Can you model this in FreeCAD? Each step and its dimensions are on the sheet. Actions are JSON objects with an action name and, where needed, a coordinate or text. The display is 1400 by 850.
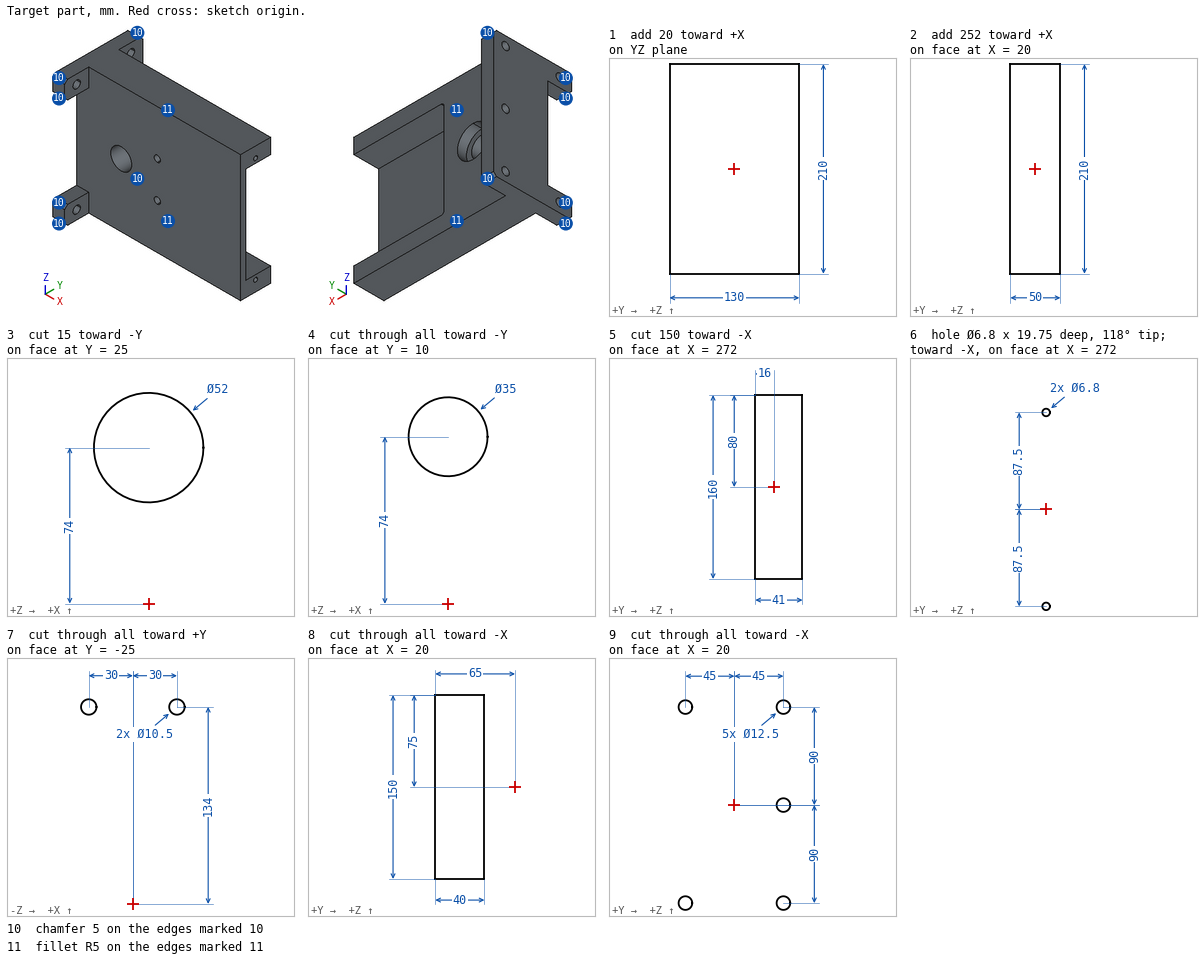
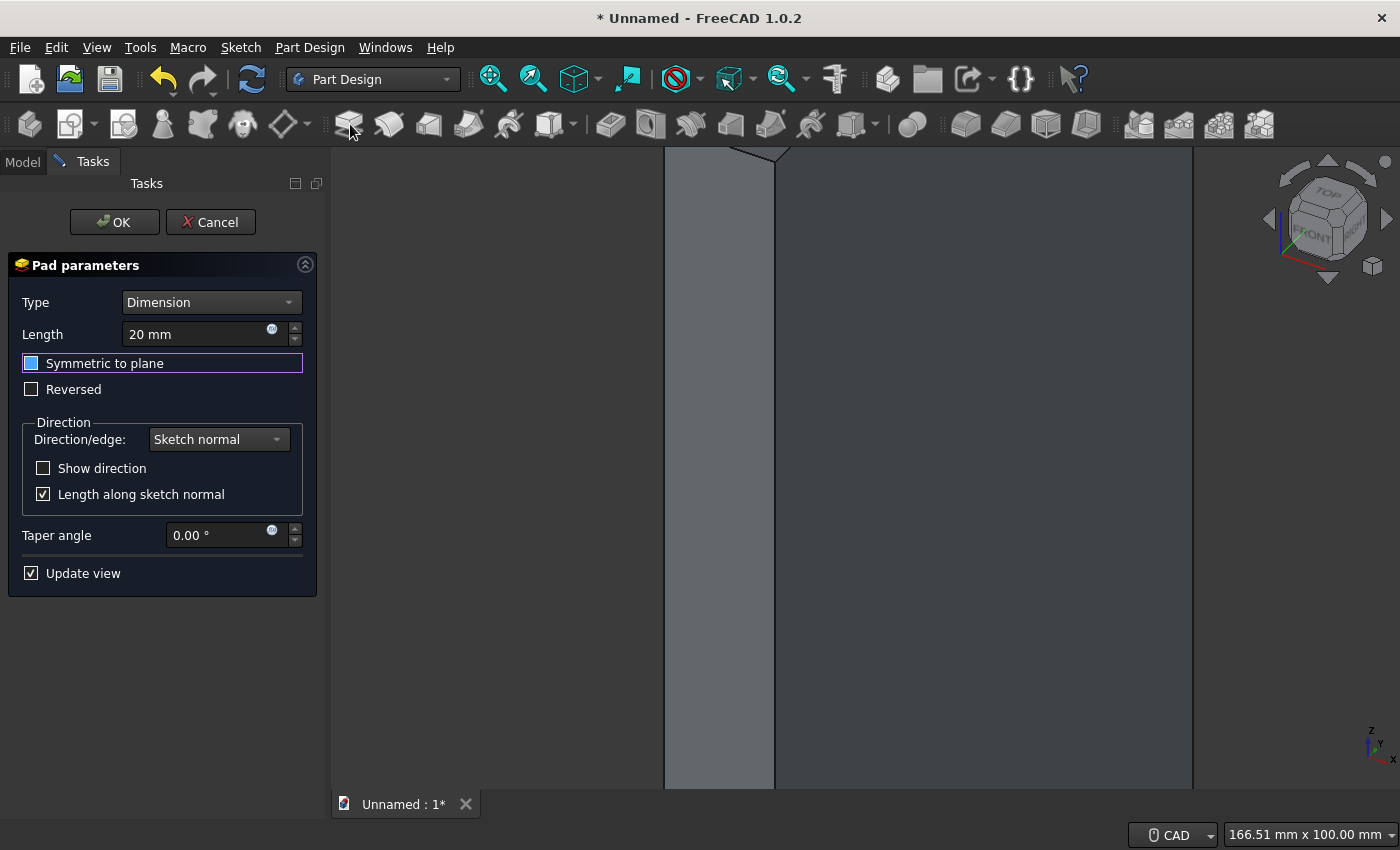
{"action": "left_click", "coordinate": [115, 222]}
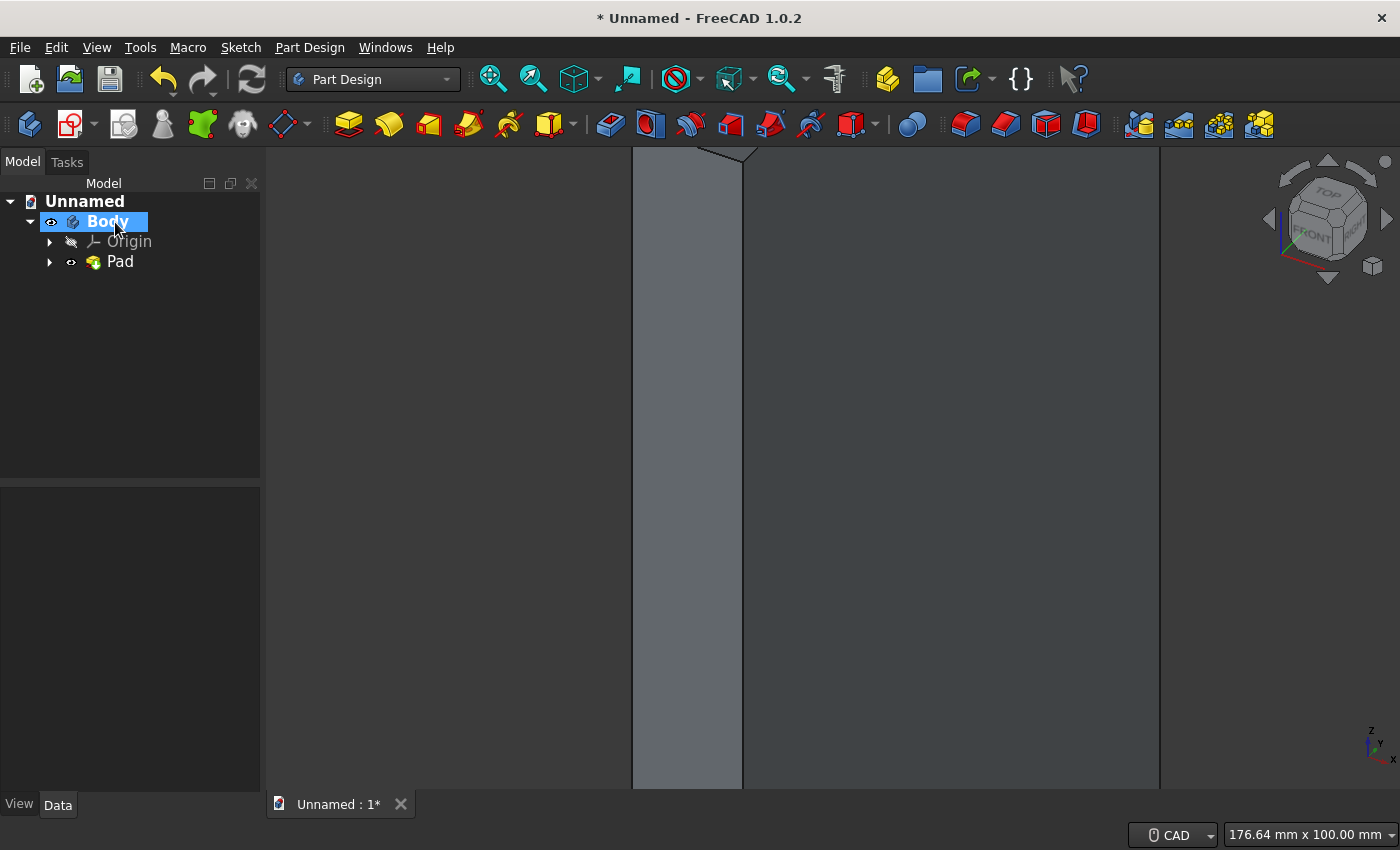
{"action": "left_click", "coordinate": [494, 80]}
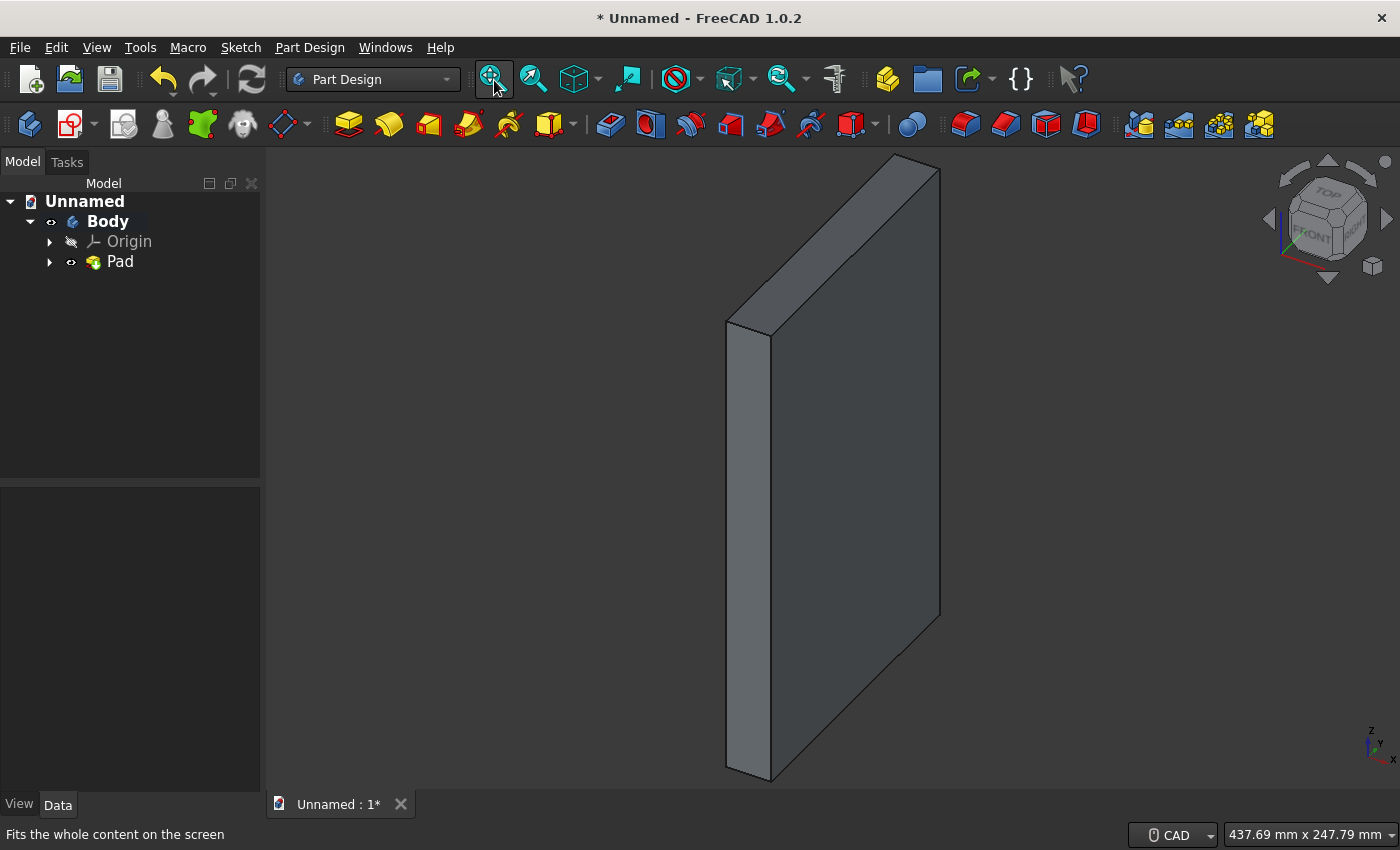
{"action": "left_click", "coordinate": [855, 474]}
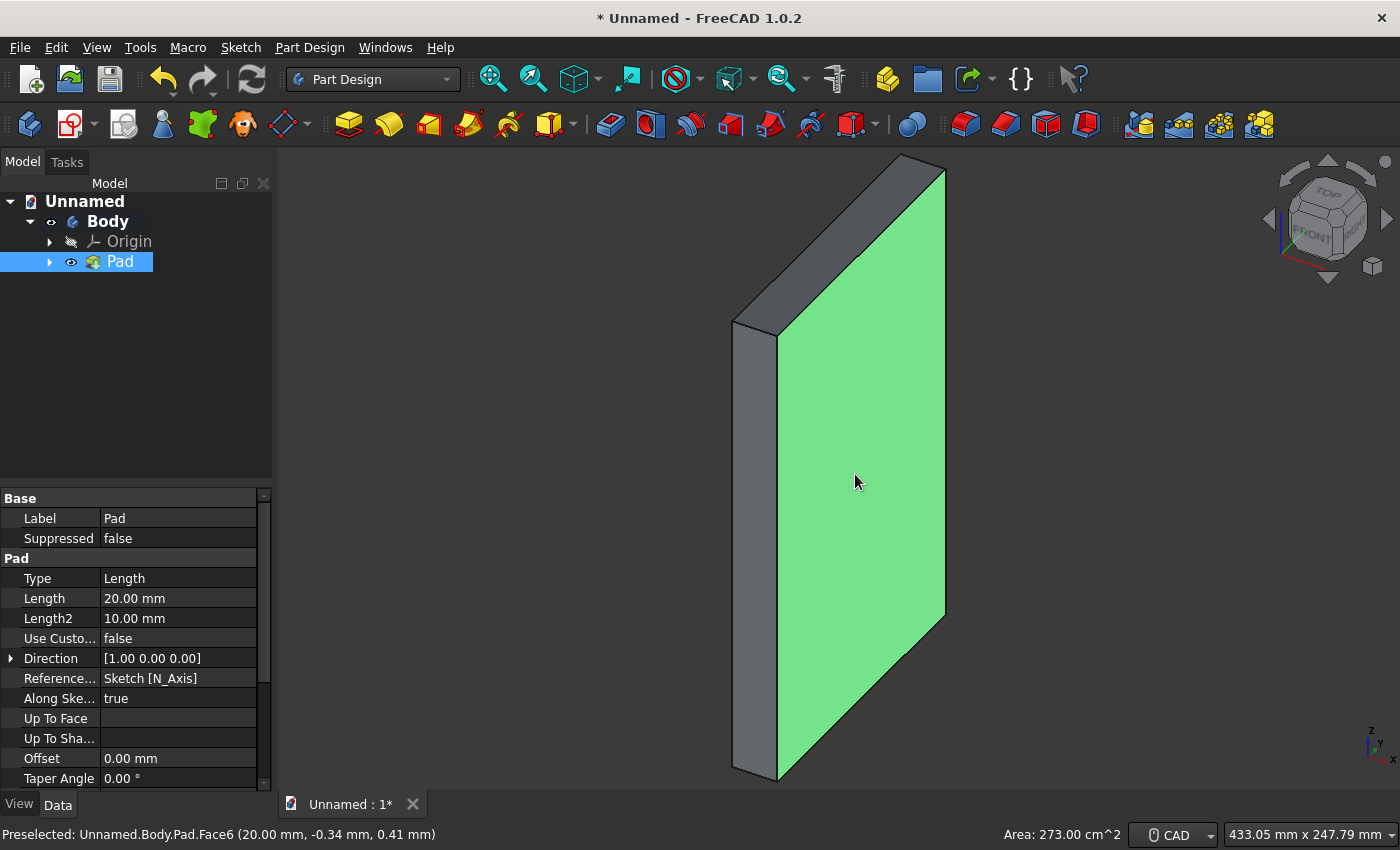
{"action": "left_click", "coordinate": [70, 124]}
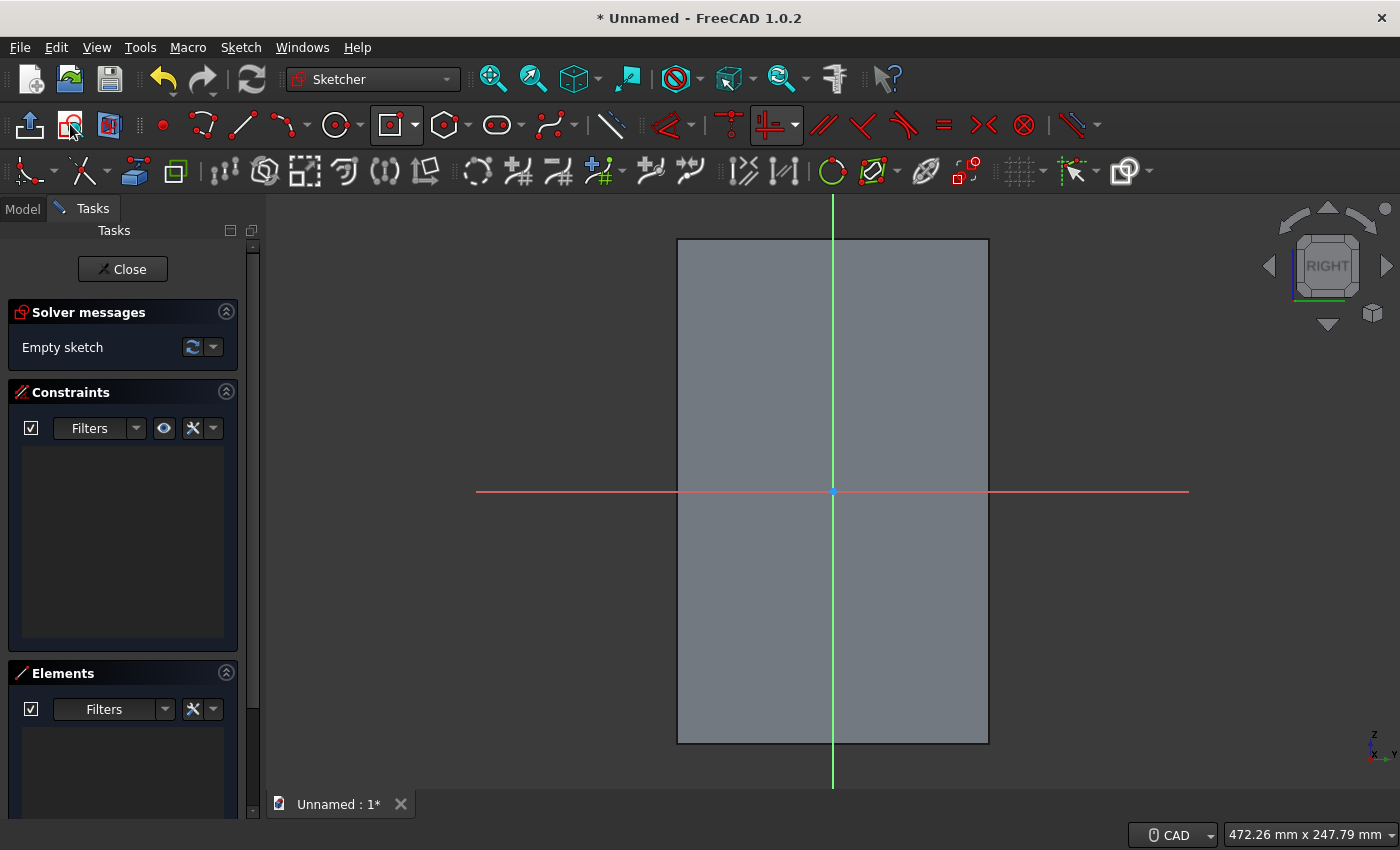
{"action": "scroll", "coordinate": [455, 492], "scroll_direction": "down", "scroll_amount": 1}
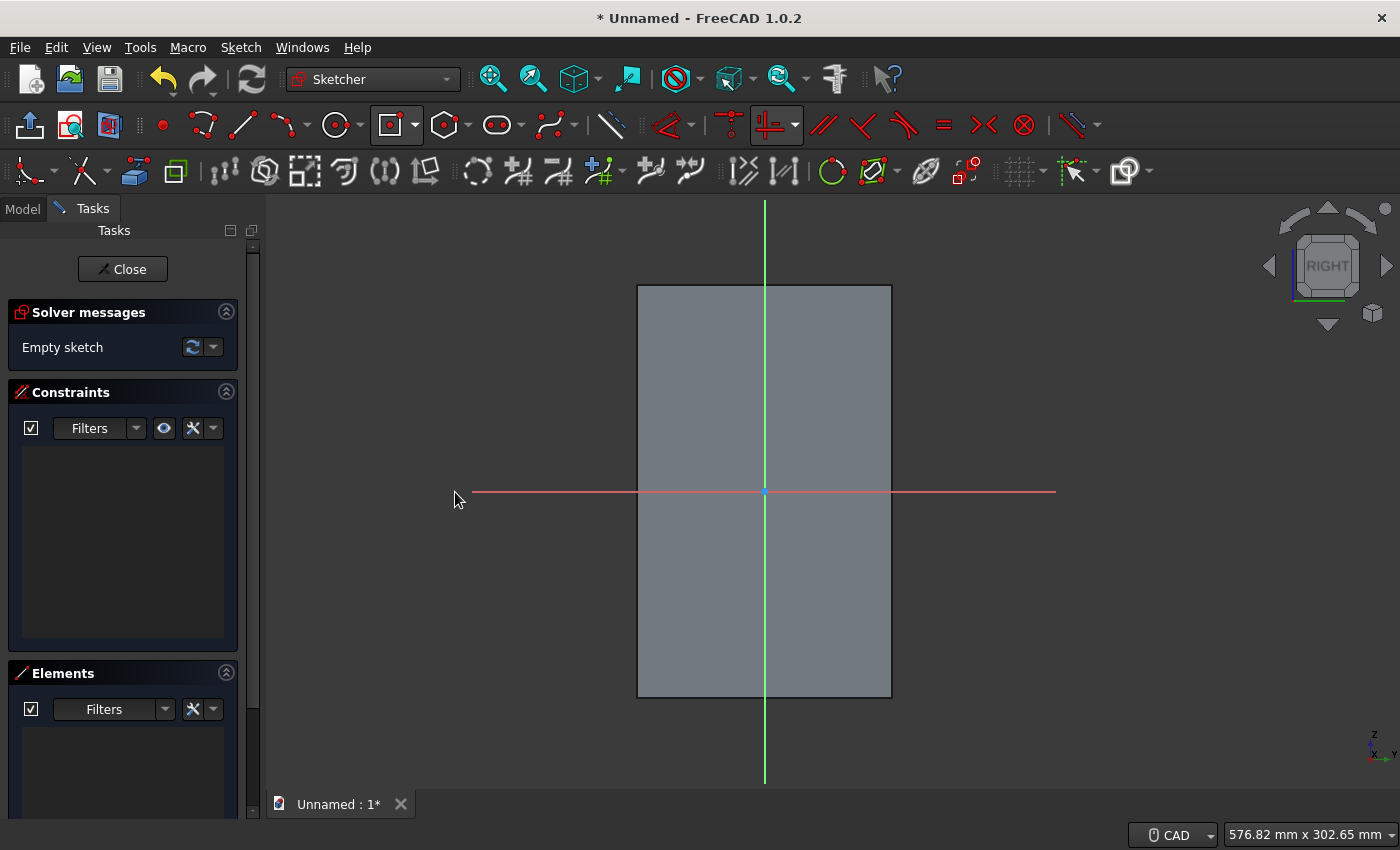
{"action": "left_click", "coordinate": [390, 126]}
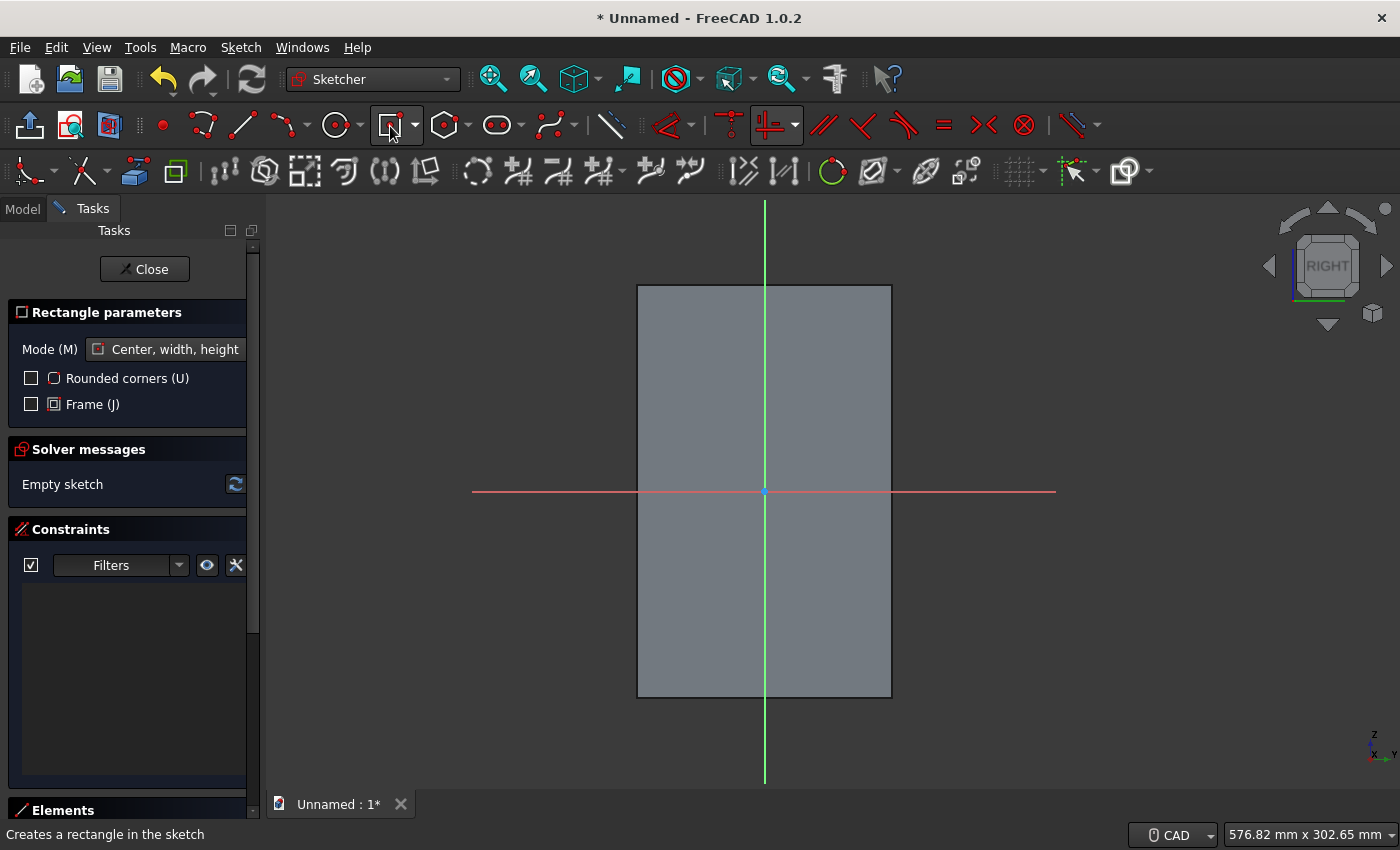
{"action": "left_click", "coordinate": [765, 492]}
{"action": "left_click", "coordinate": [814, 285]}
{"action": "key", "text": "Escape"}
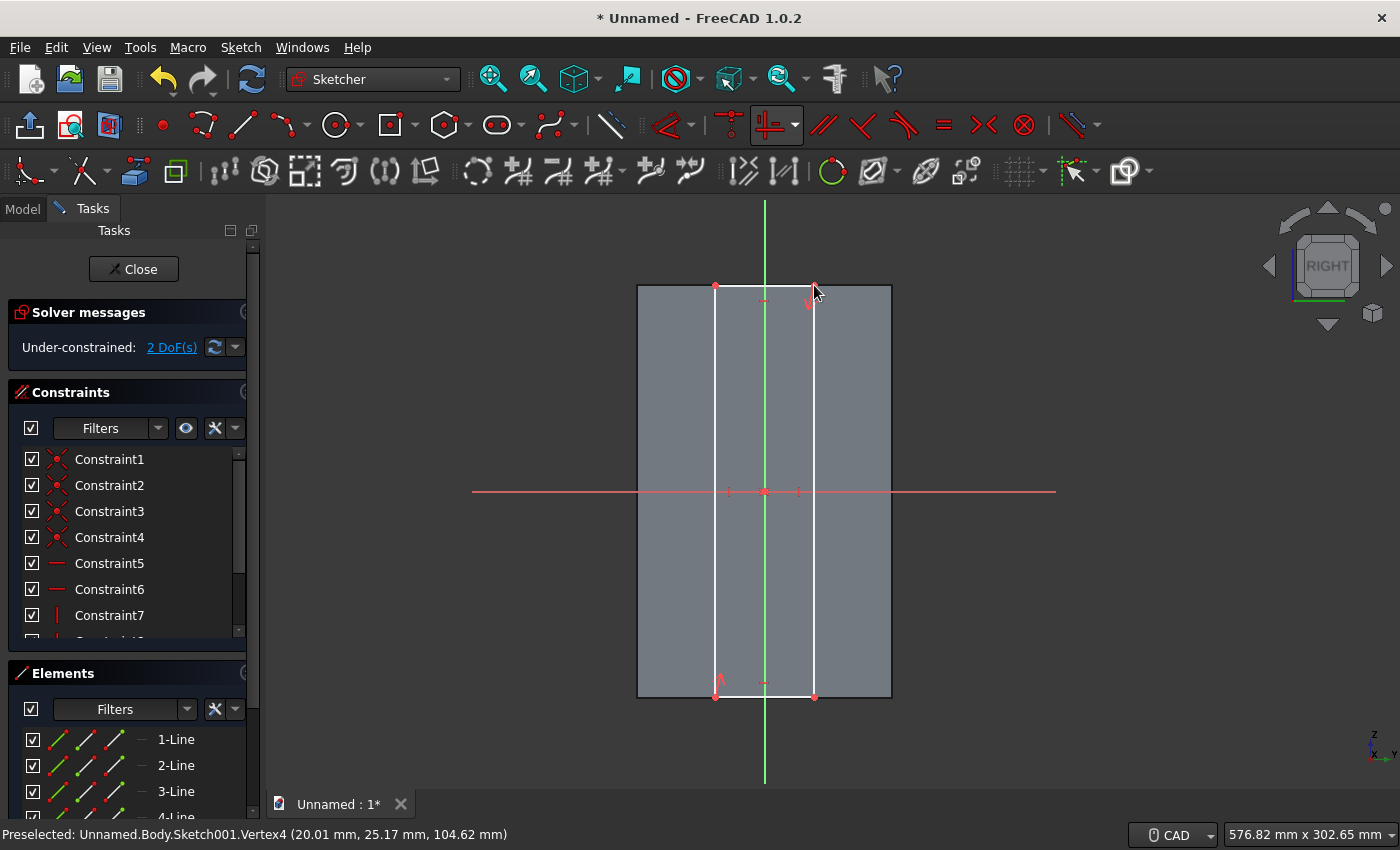
{"action": "left_click", "coordinate": [666, 126]}